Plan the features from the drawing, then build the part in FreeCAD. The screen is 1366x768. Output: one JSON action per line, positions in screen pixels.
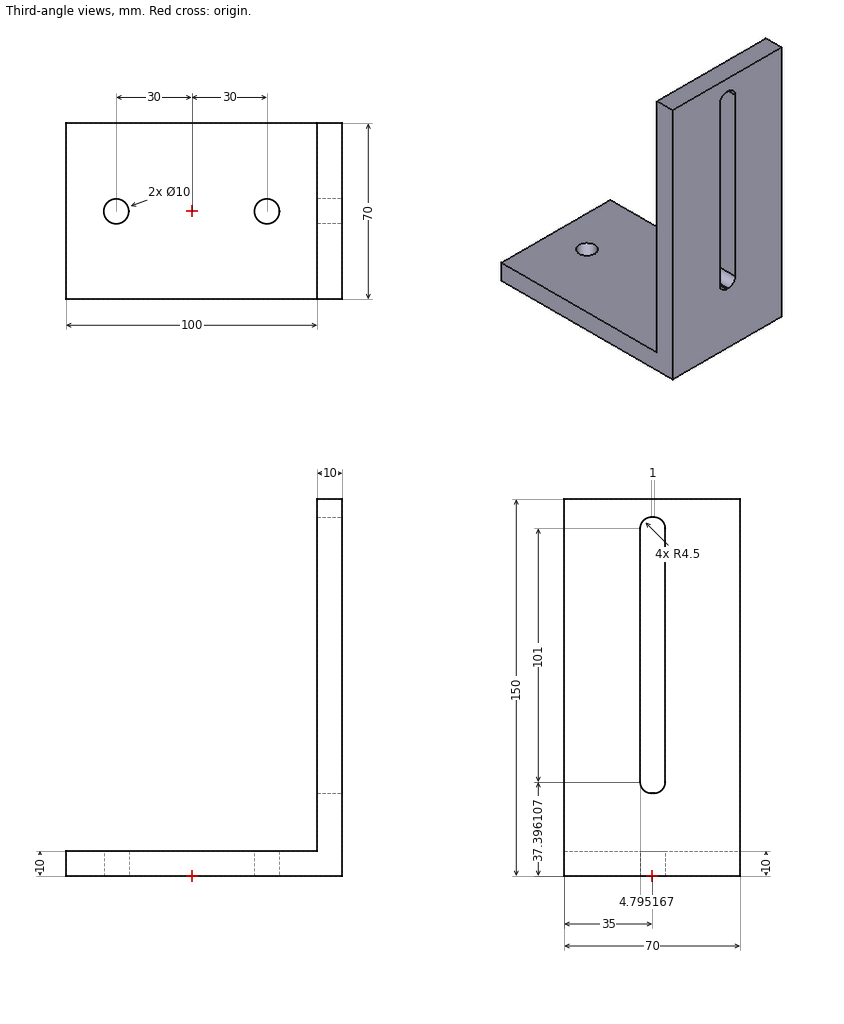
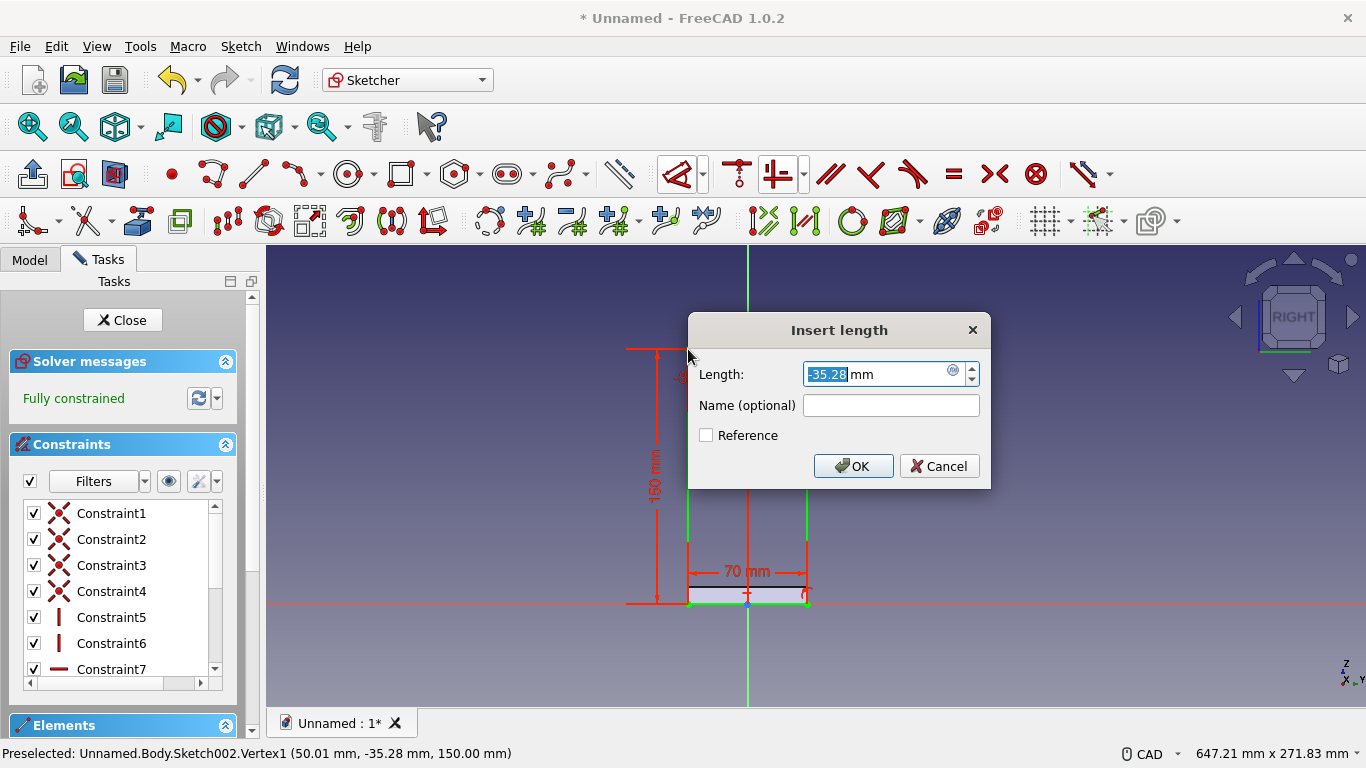
{"action": "type", "text": "-35"}
{"action": "key", "text": "Return"}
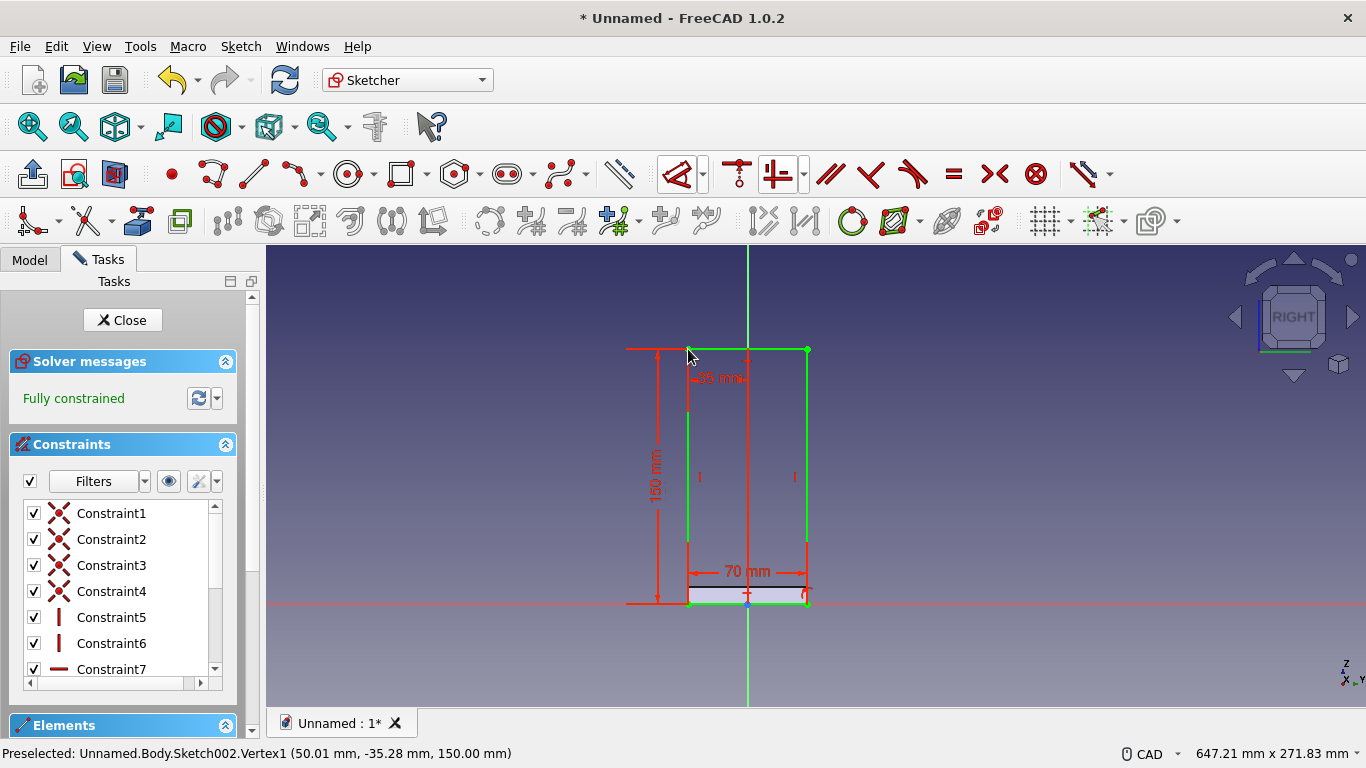
{"action": "left_click", "coordinate": [123, 320]}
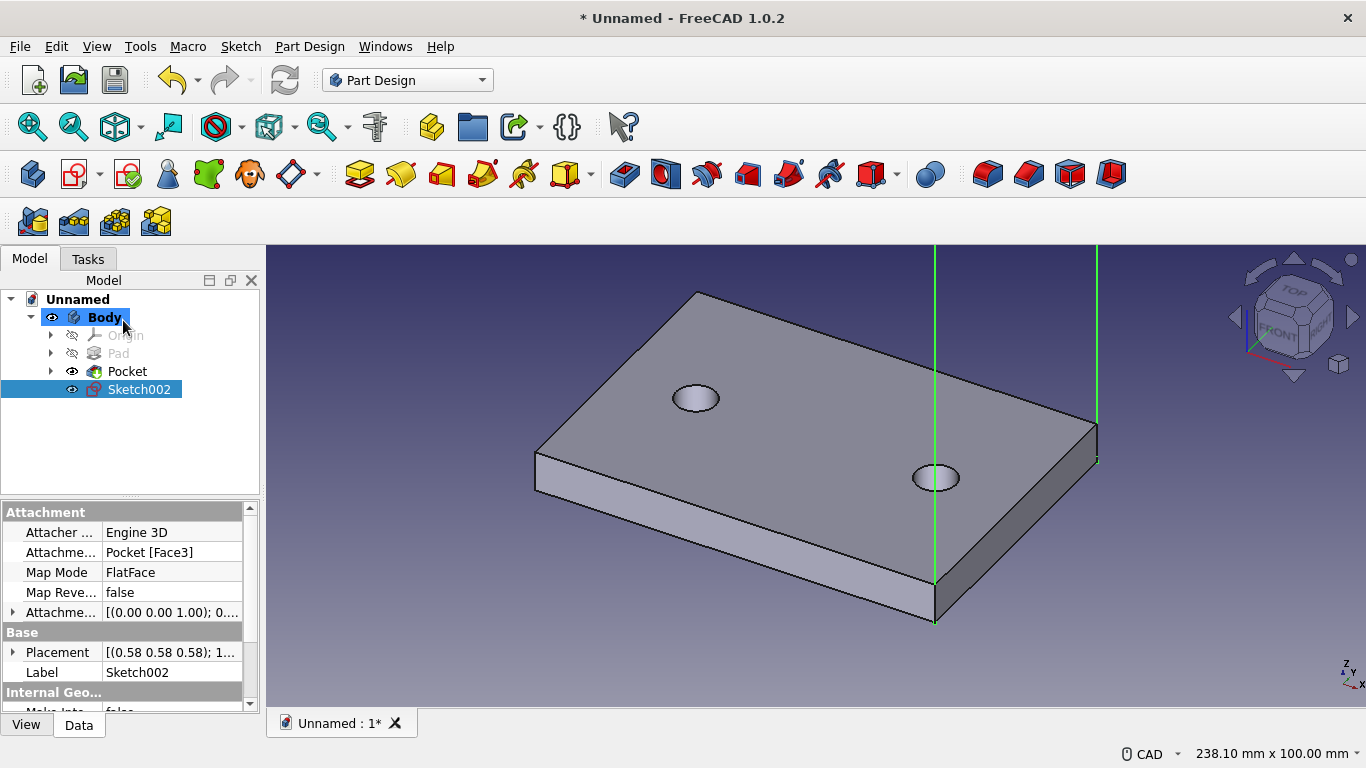
{"action": "left_click", "coordinate": [360, 174]}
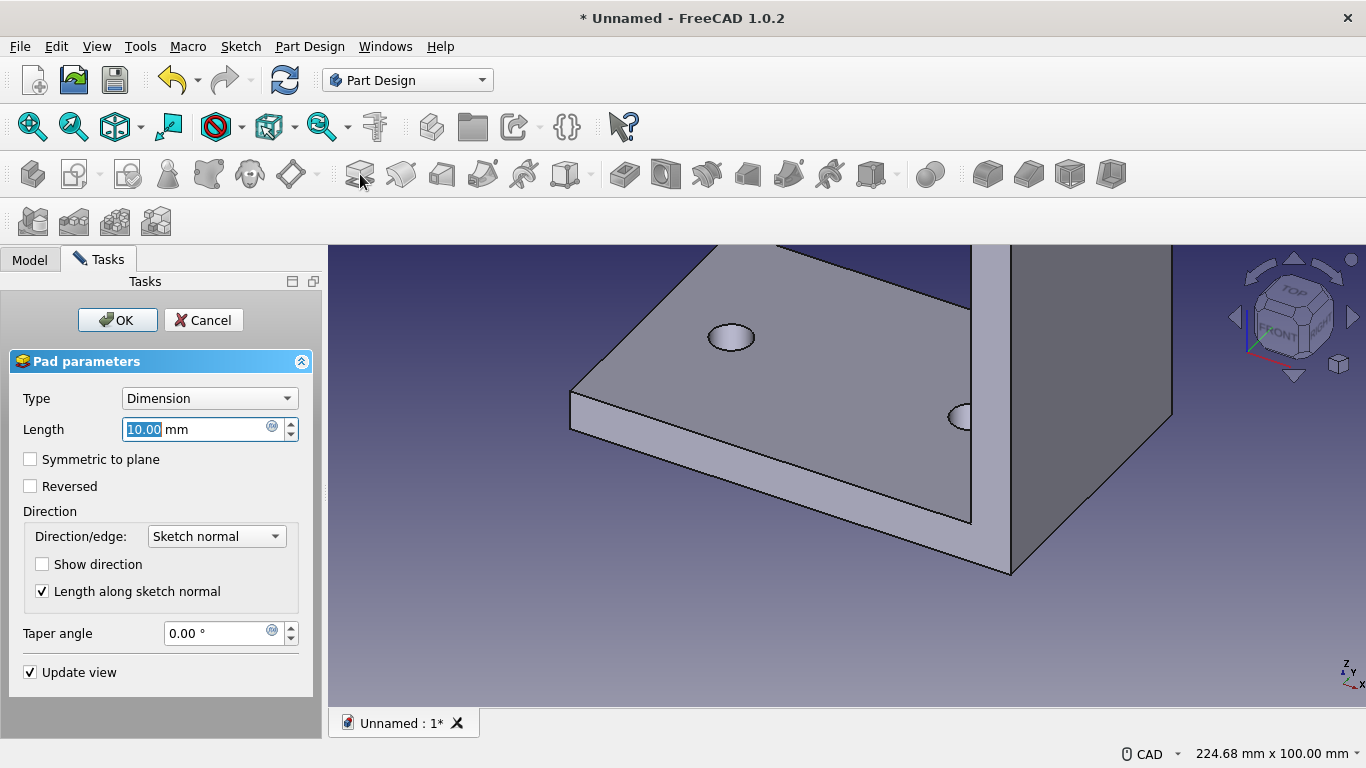
{"action": "type", "text": "10"}
{"action": "key", "text": "Tab"}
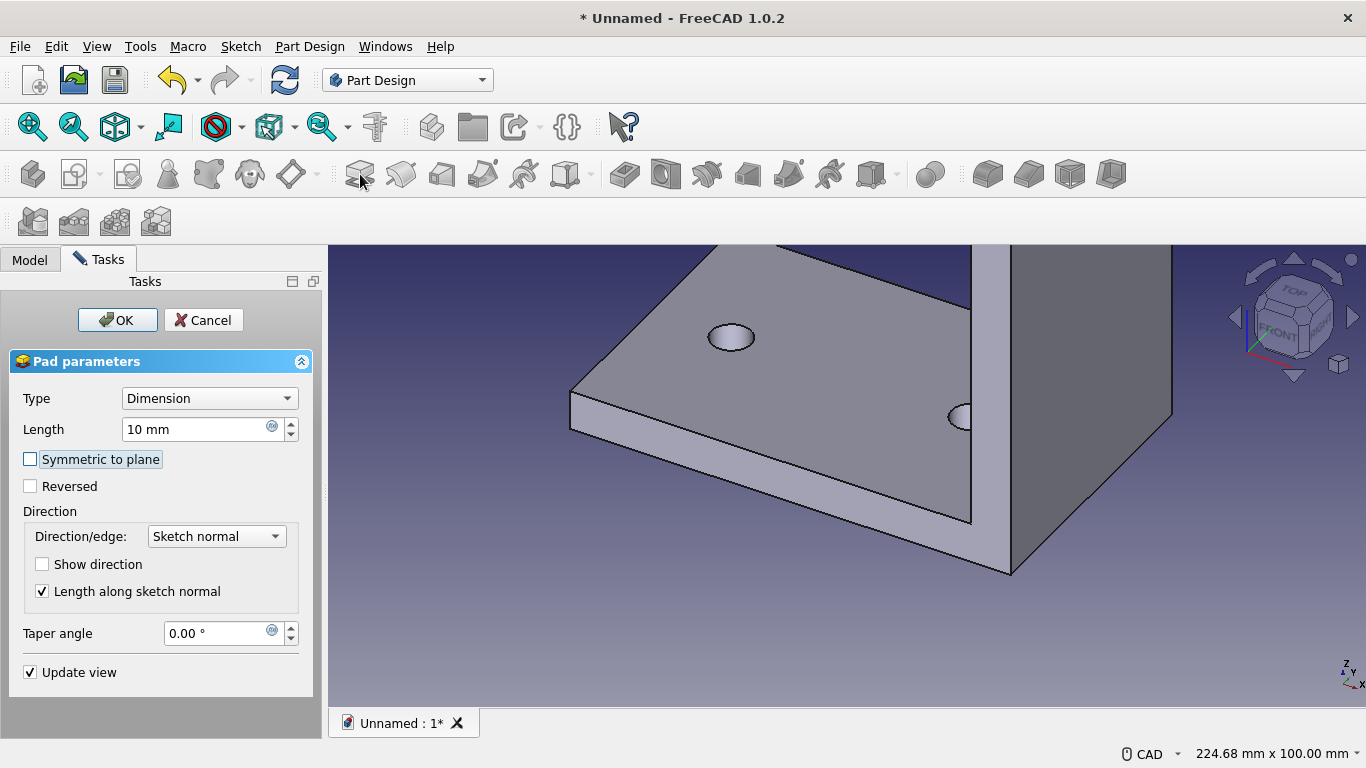
{"action": "left_click", "coordinate": [118, 320]}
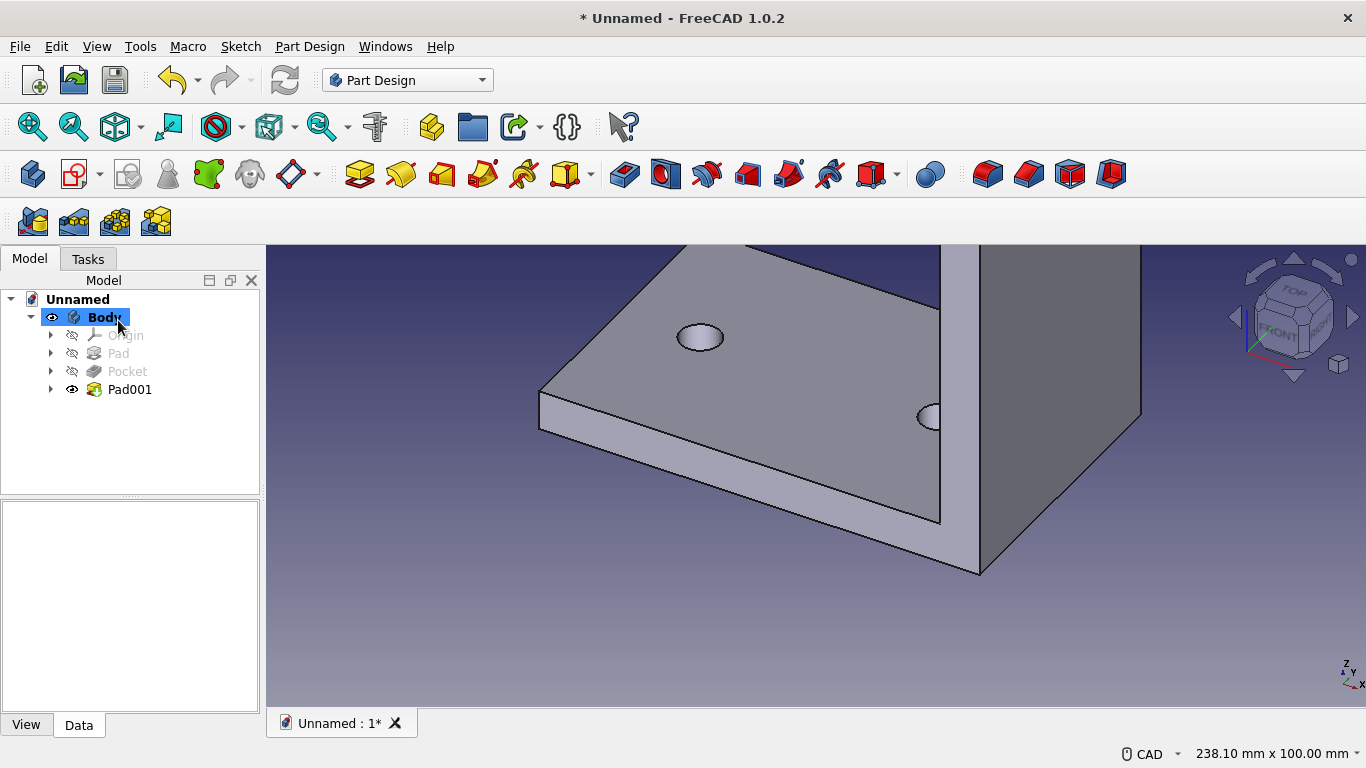
{"action": "left_click", "coordinate": [33, 128]}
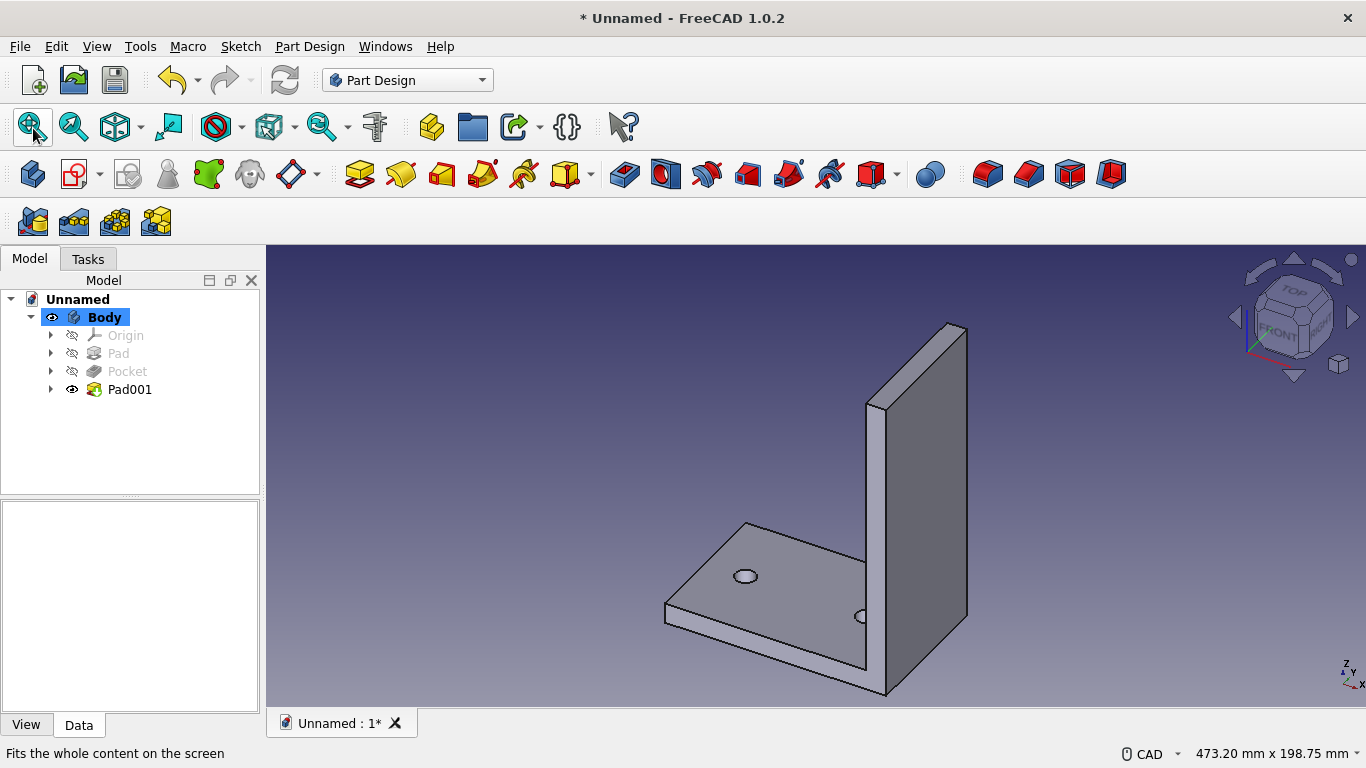
{"action": "key", "text": "6"}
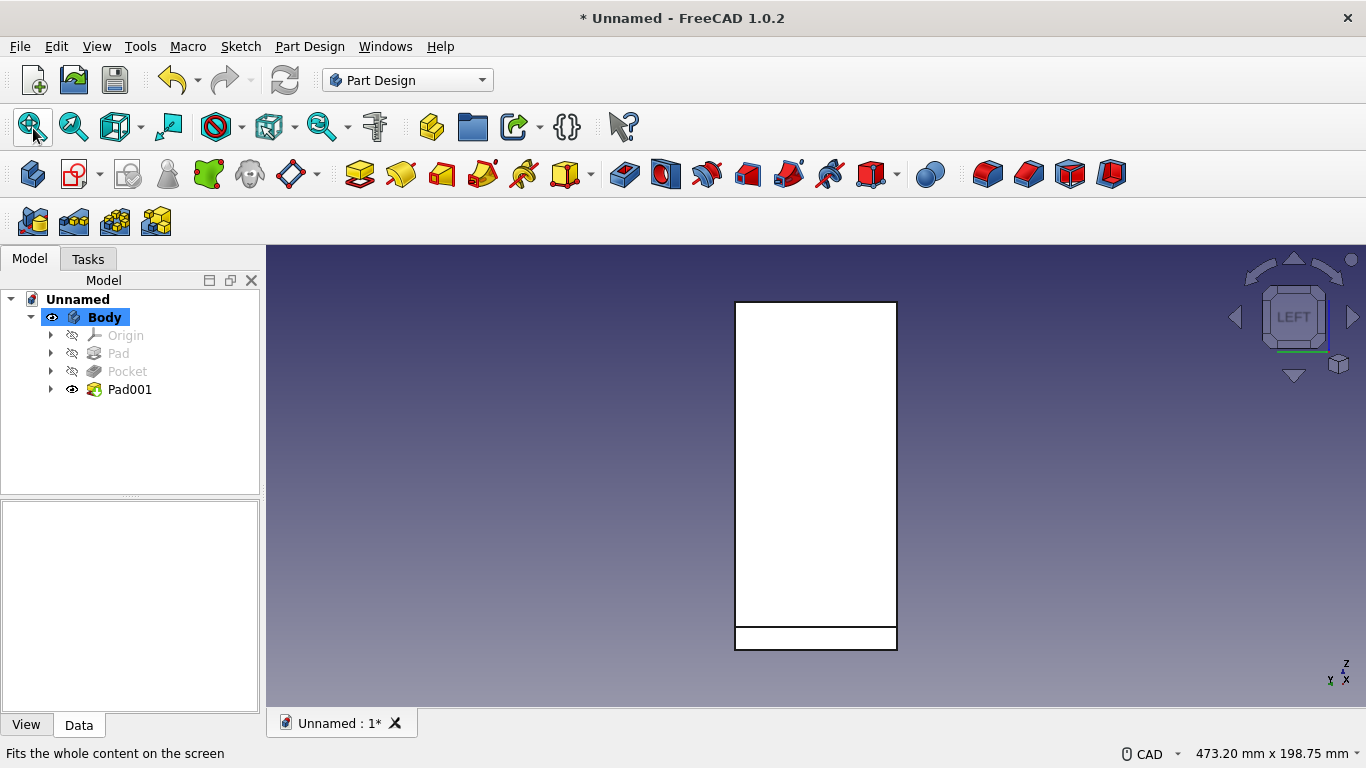
{"action": "left_click", "coordinate": [816, 417]}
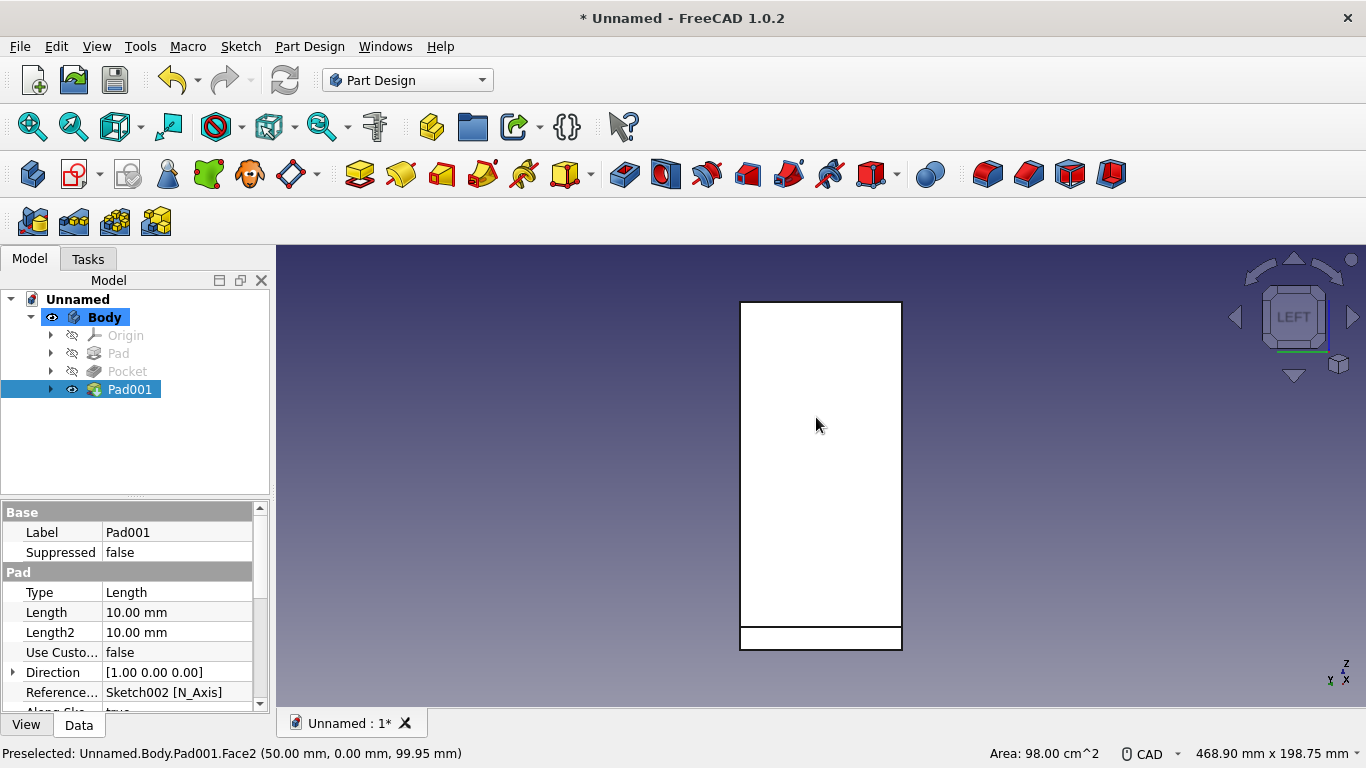
{"action": "left_click", "coordinate": [74, 174]}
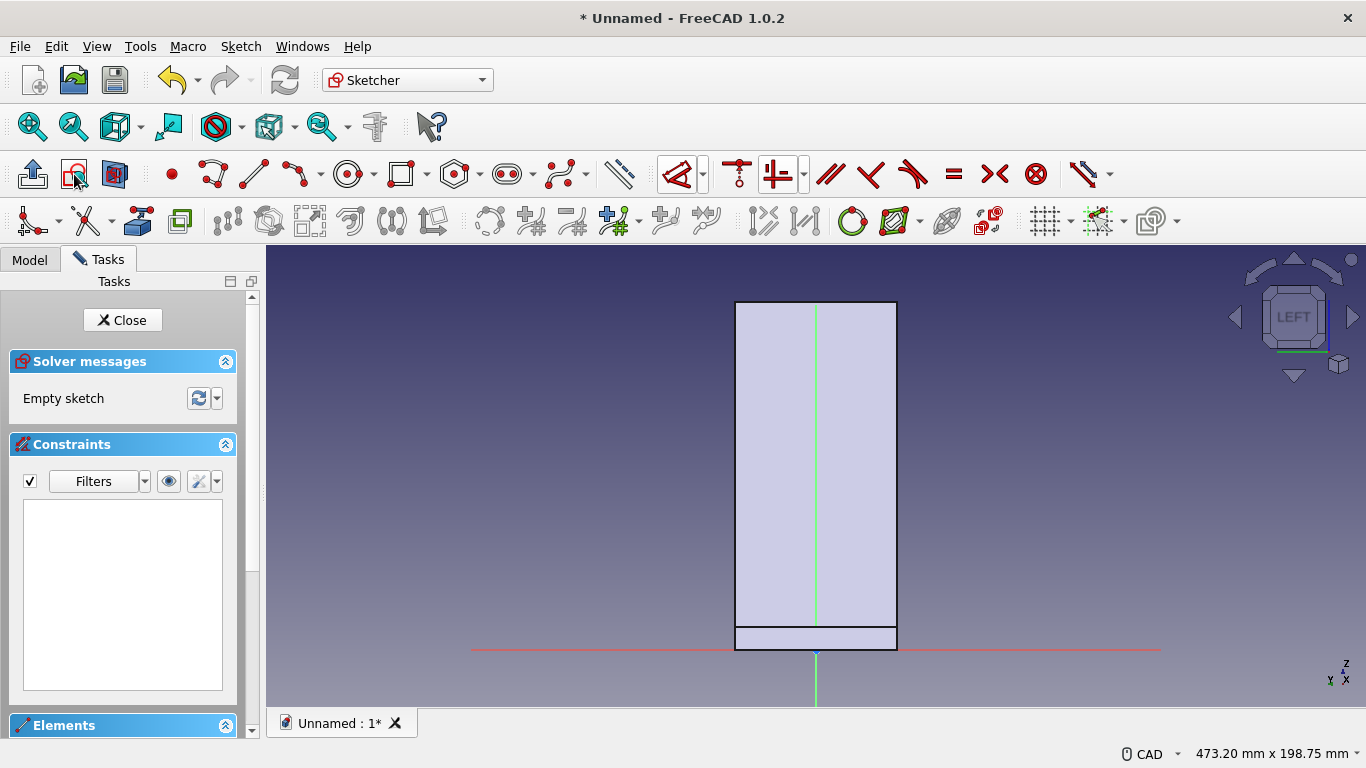
{"action": "left_click", "coordinate": [254, 174]}